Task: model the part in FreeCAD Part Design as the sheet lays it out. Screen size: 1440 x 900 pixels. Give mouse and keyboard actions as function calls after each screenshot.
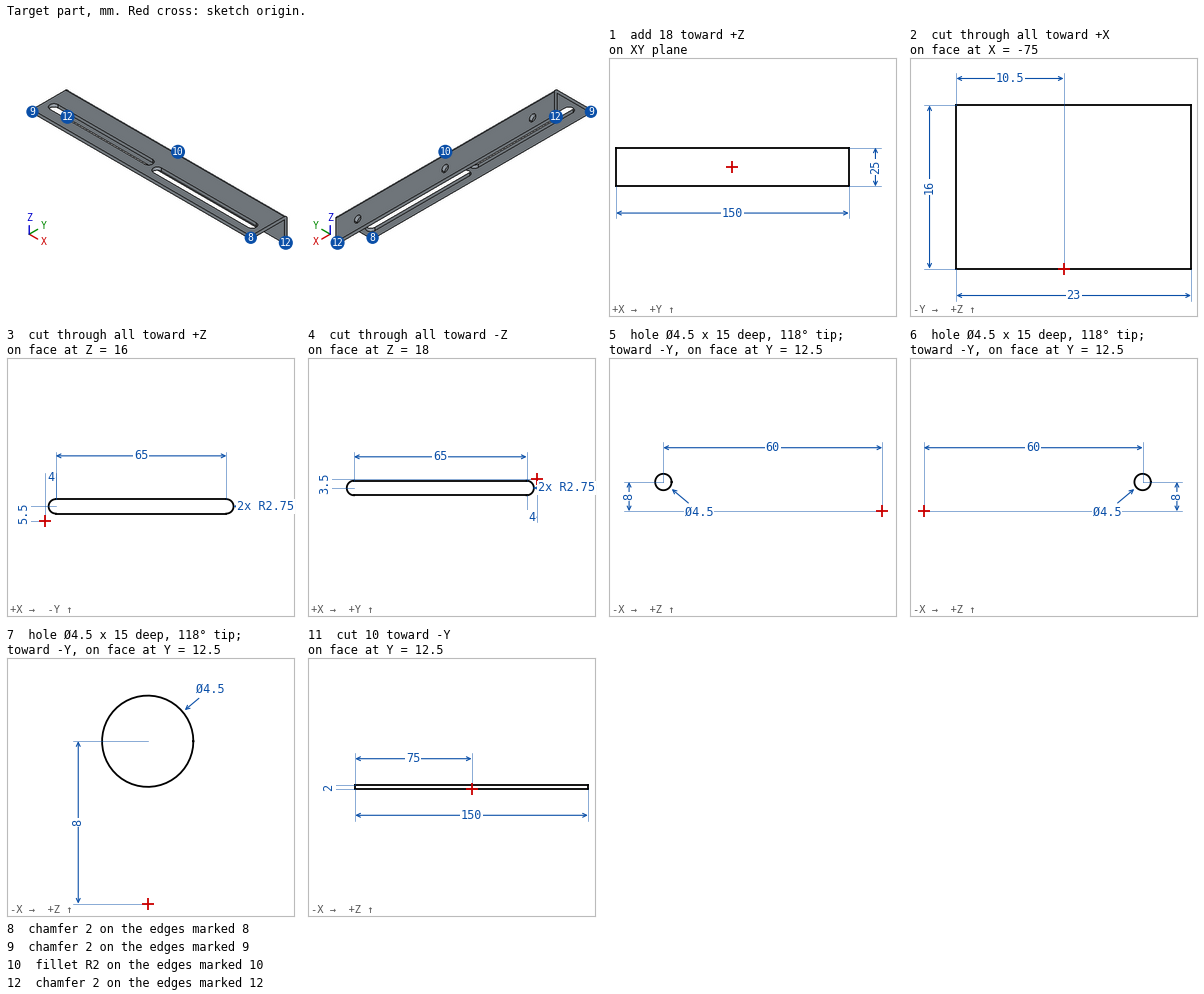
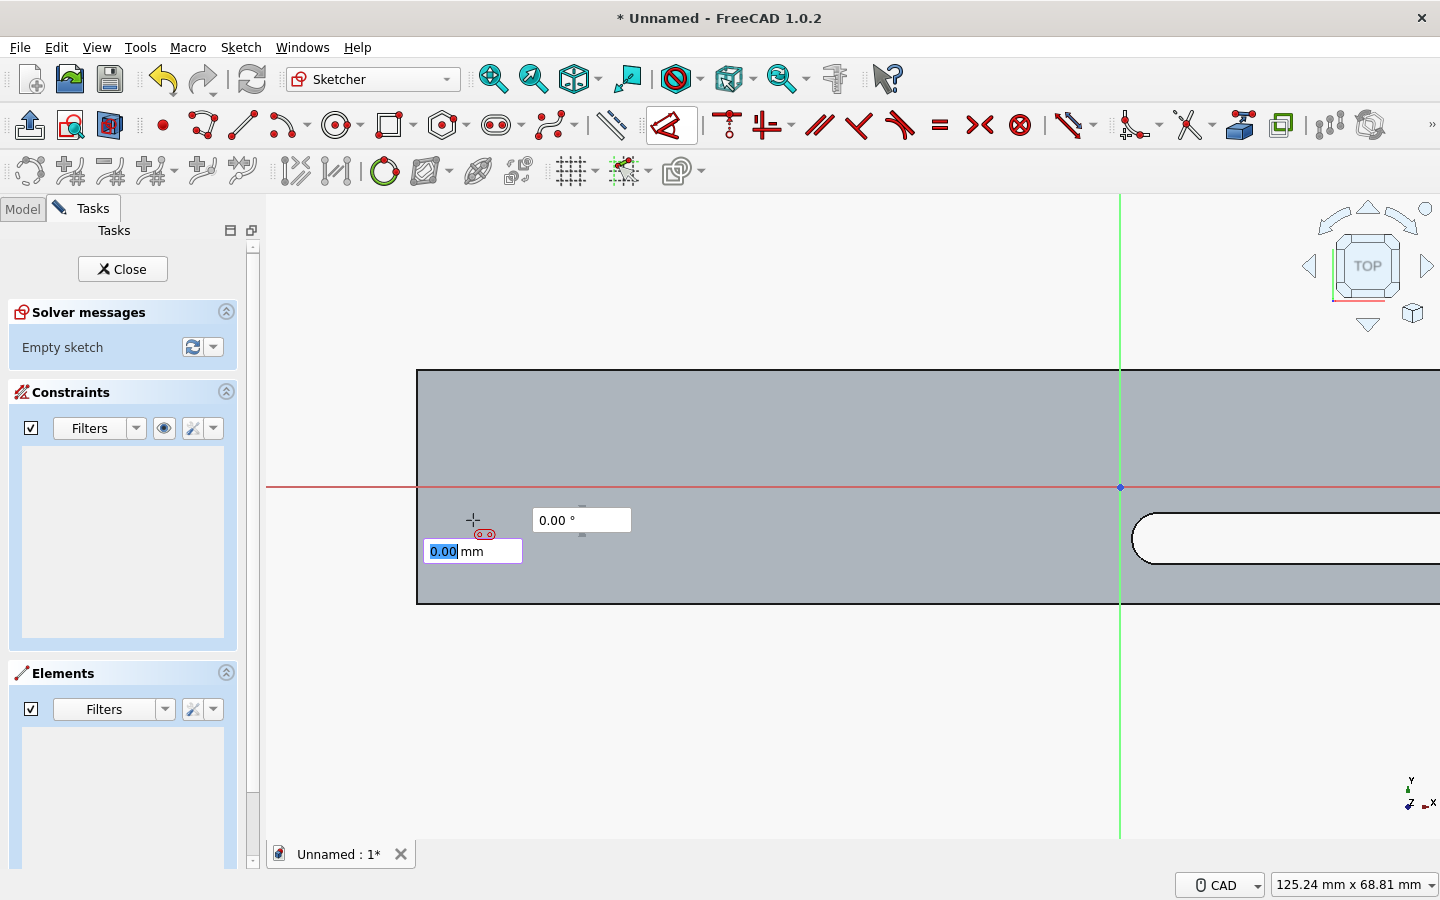
click(1083, 520)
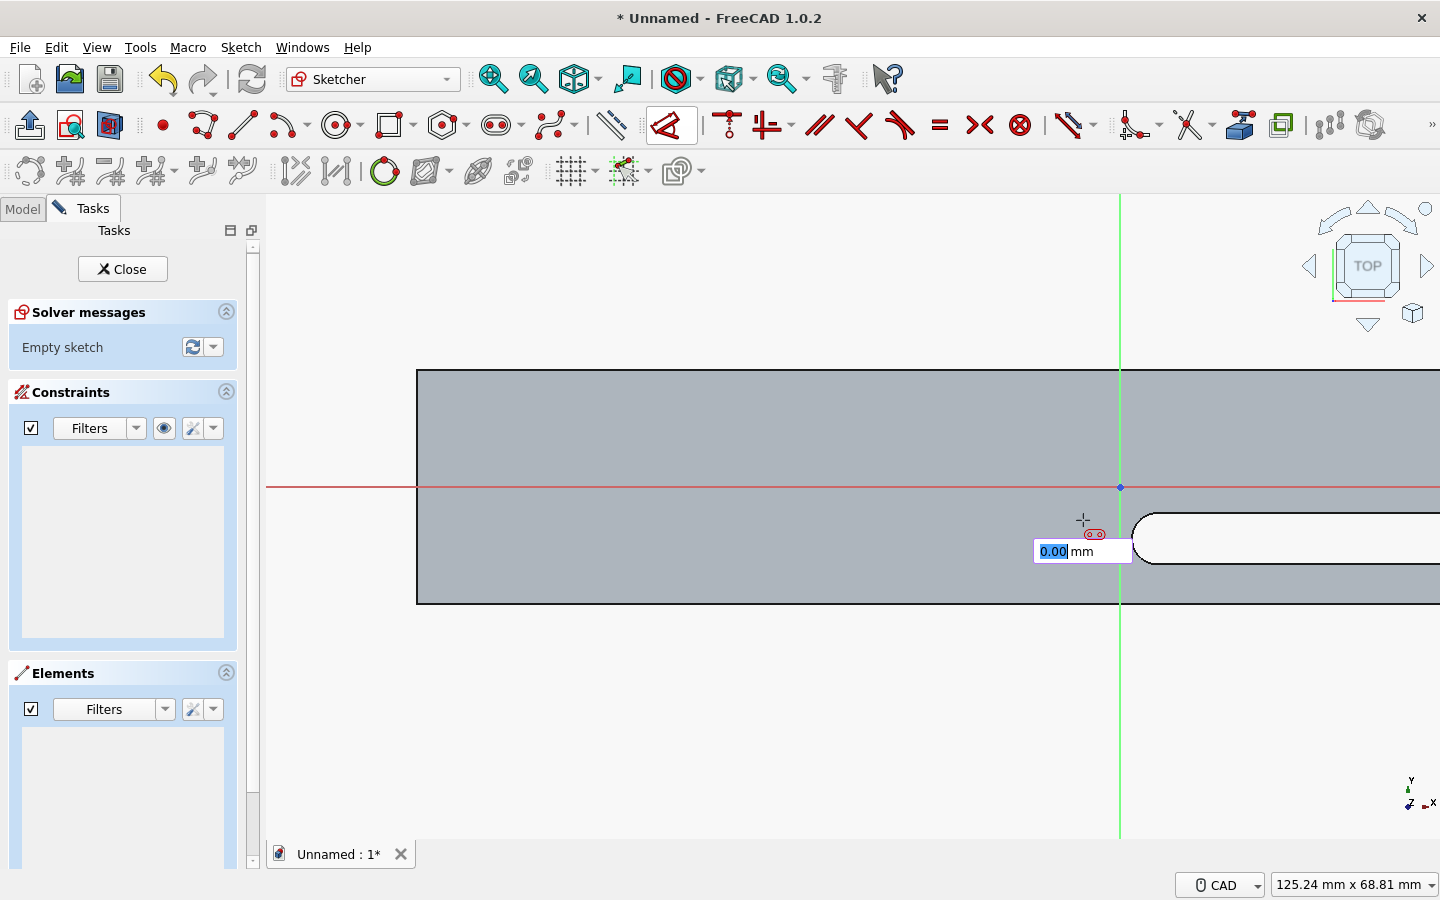
click(778, 546)
key(Escape)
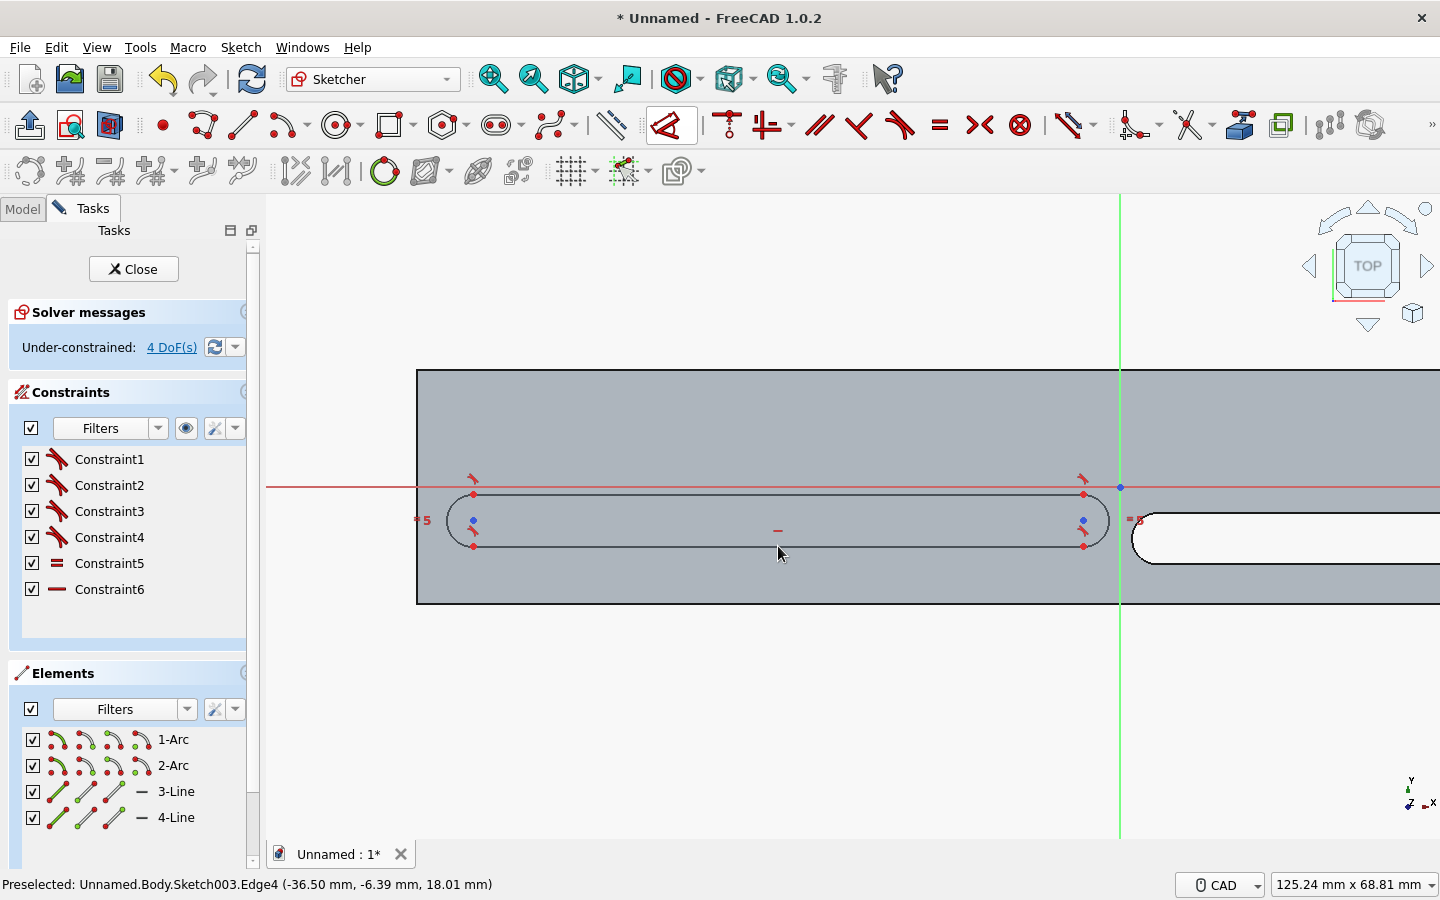
scroll(452, 506, up, 3)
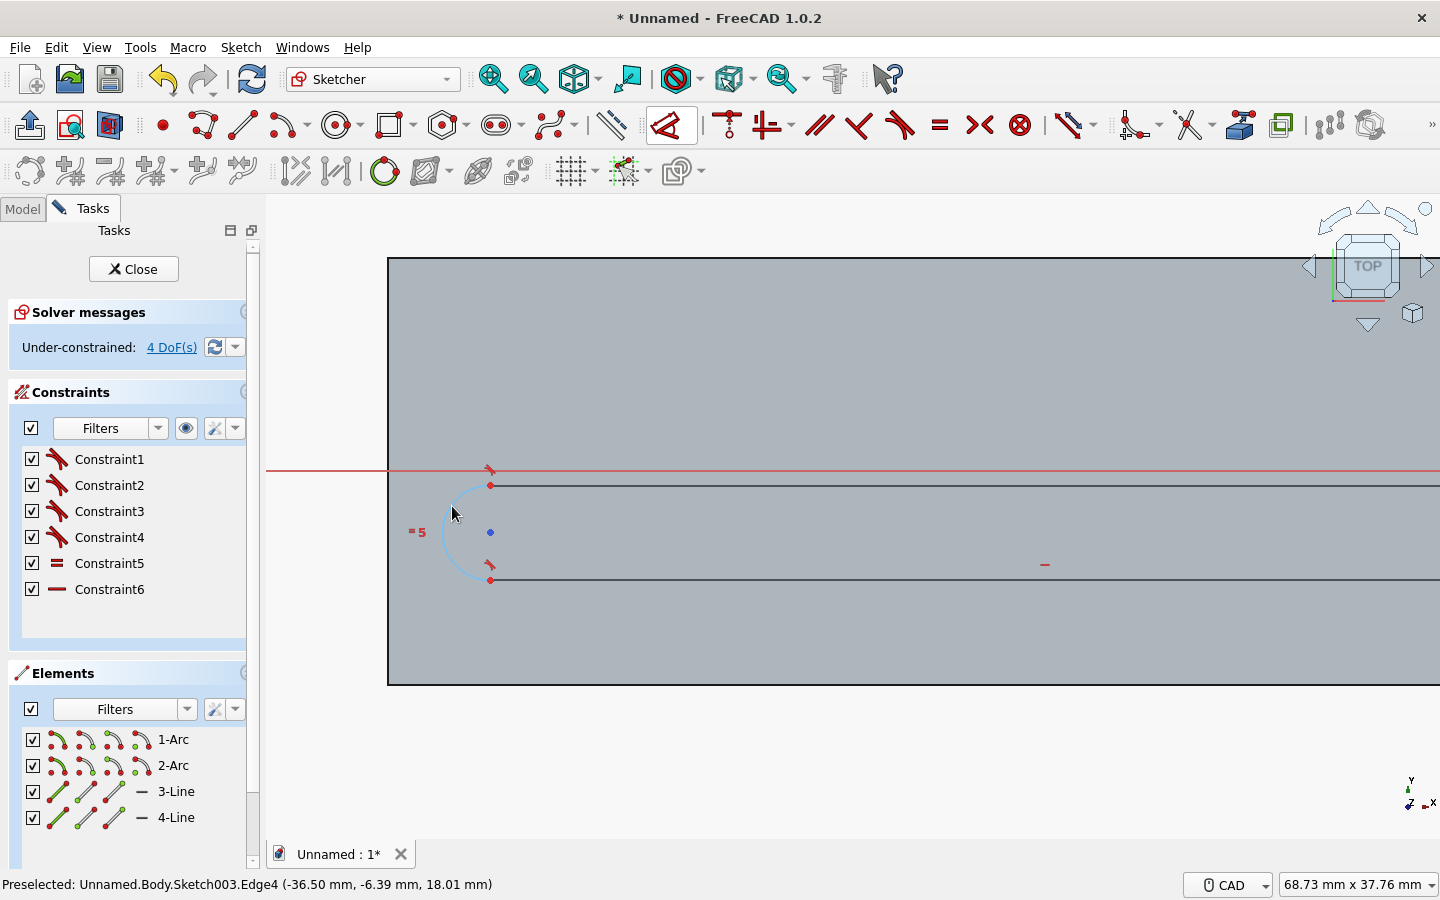
click(452, 505)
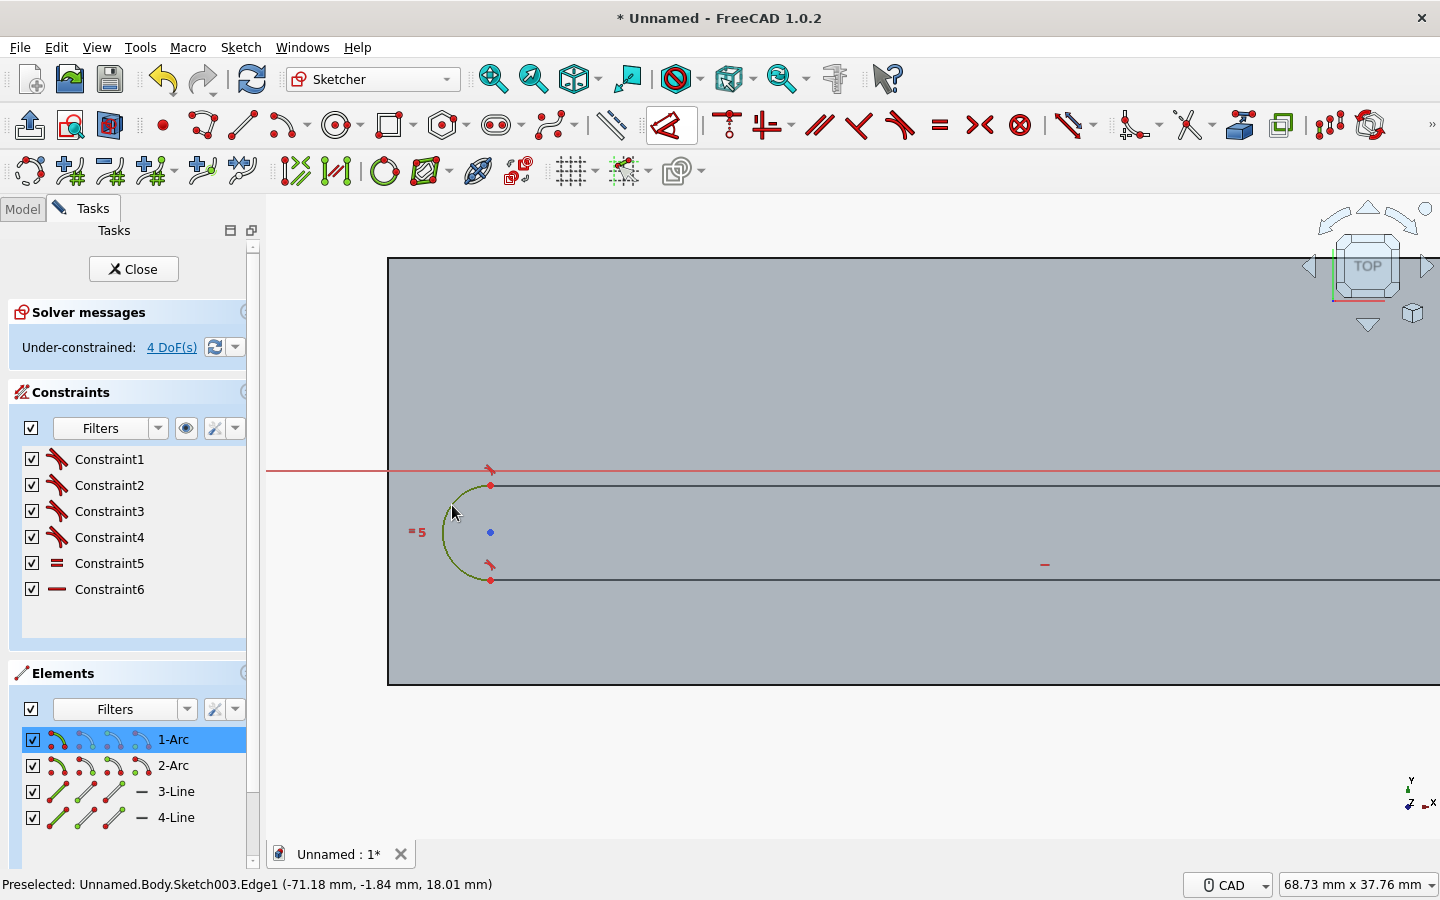
key(k)
key(r)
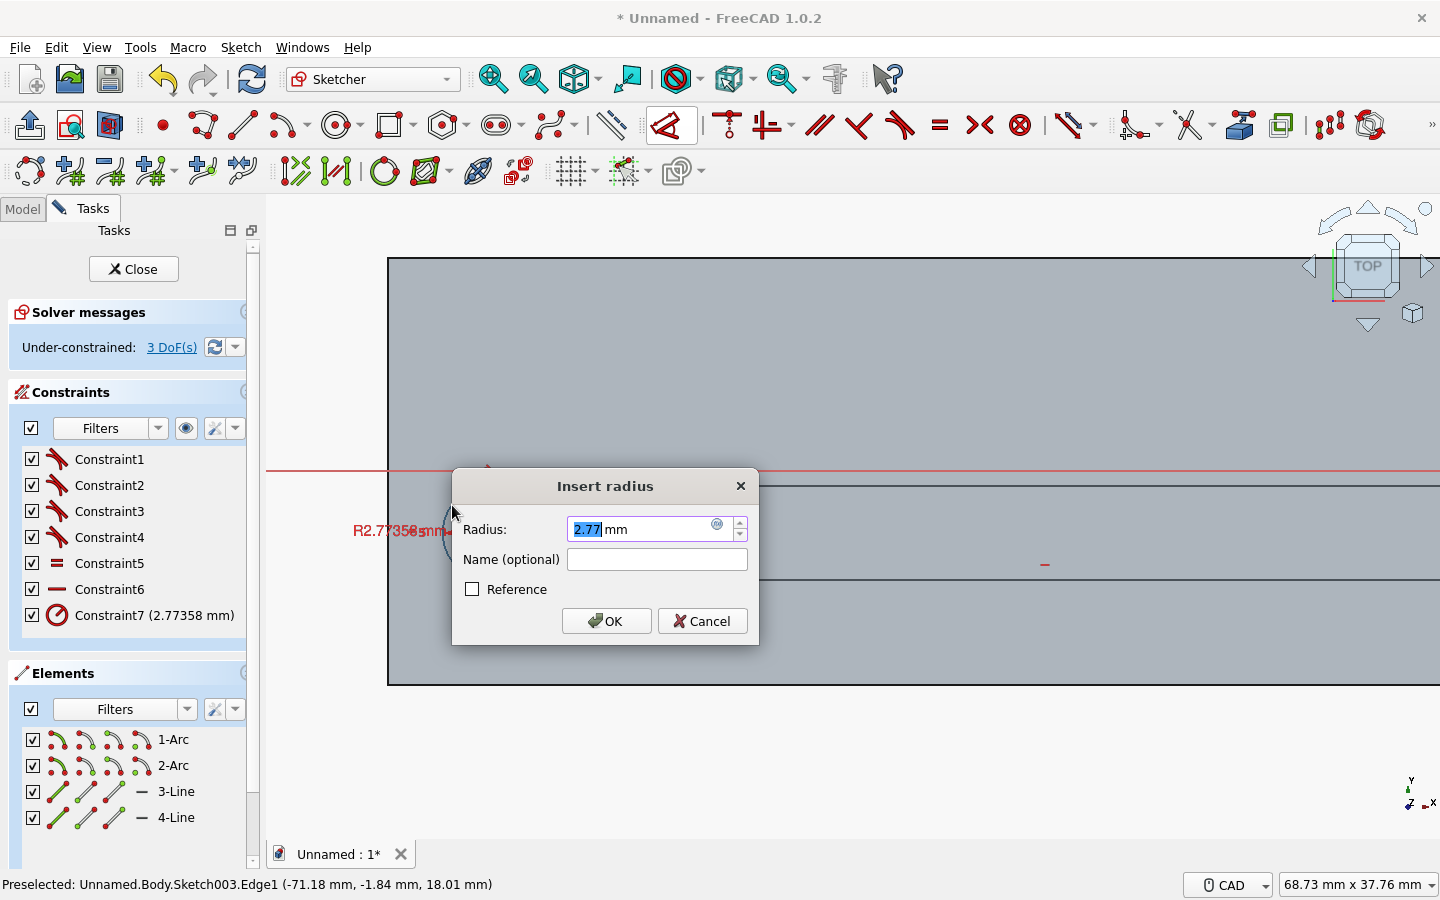
text(2.75)
key(Return)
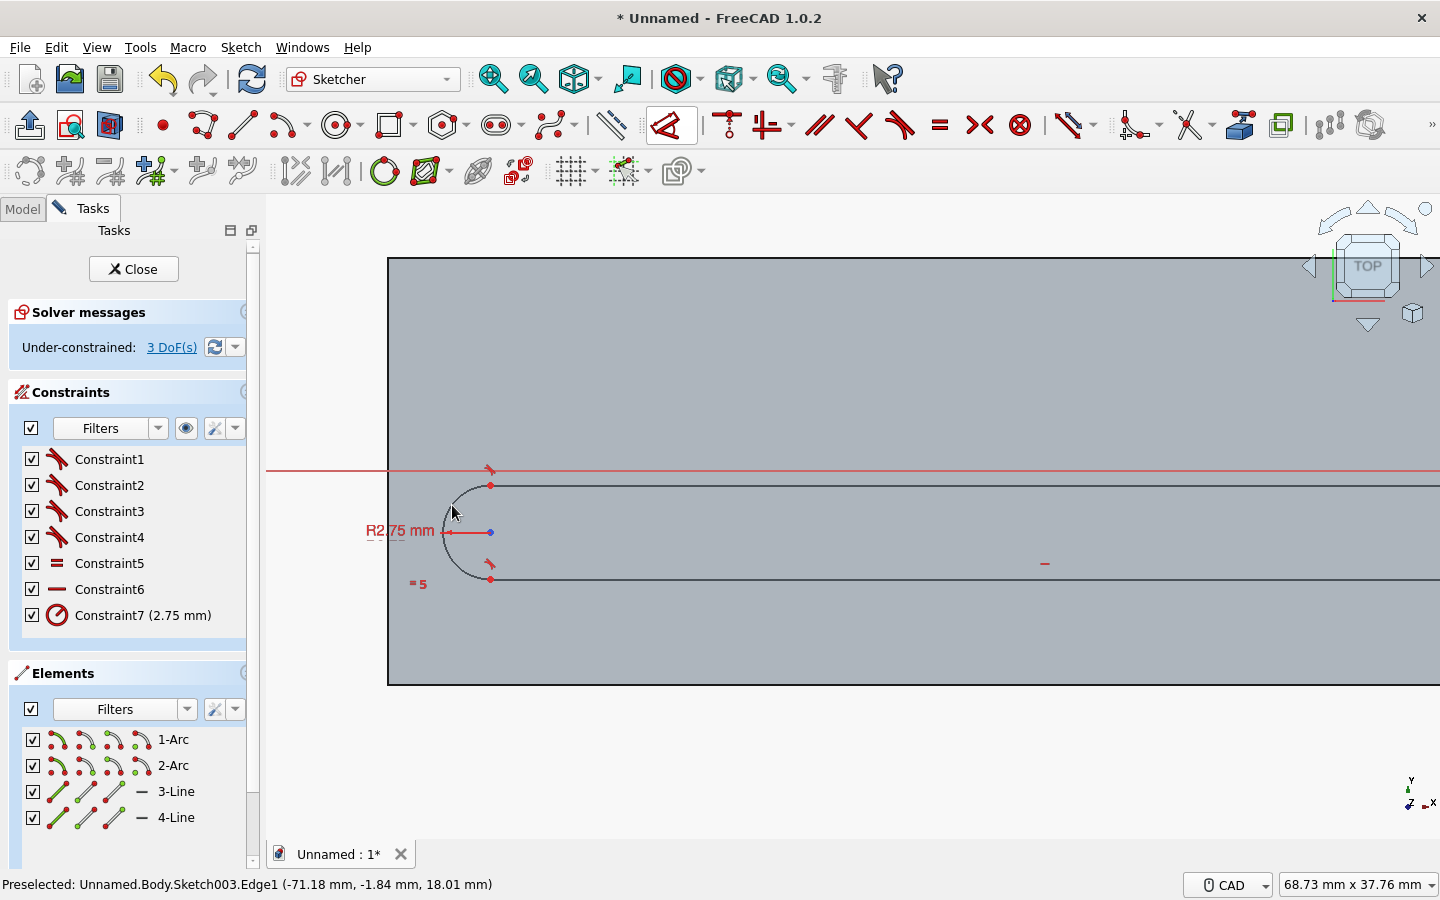
click(824, 486)